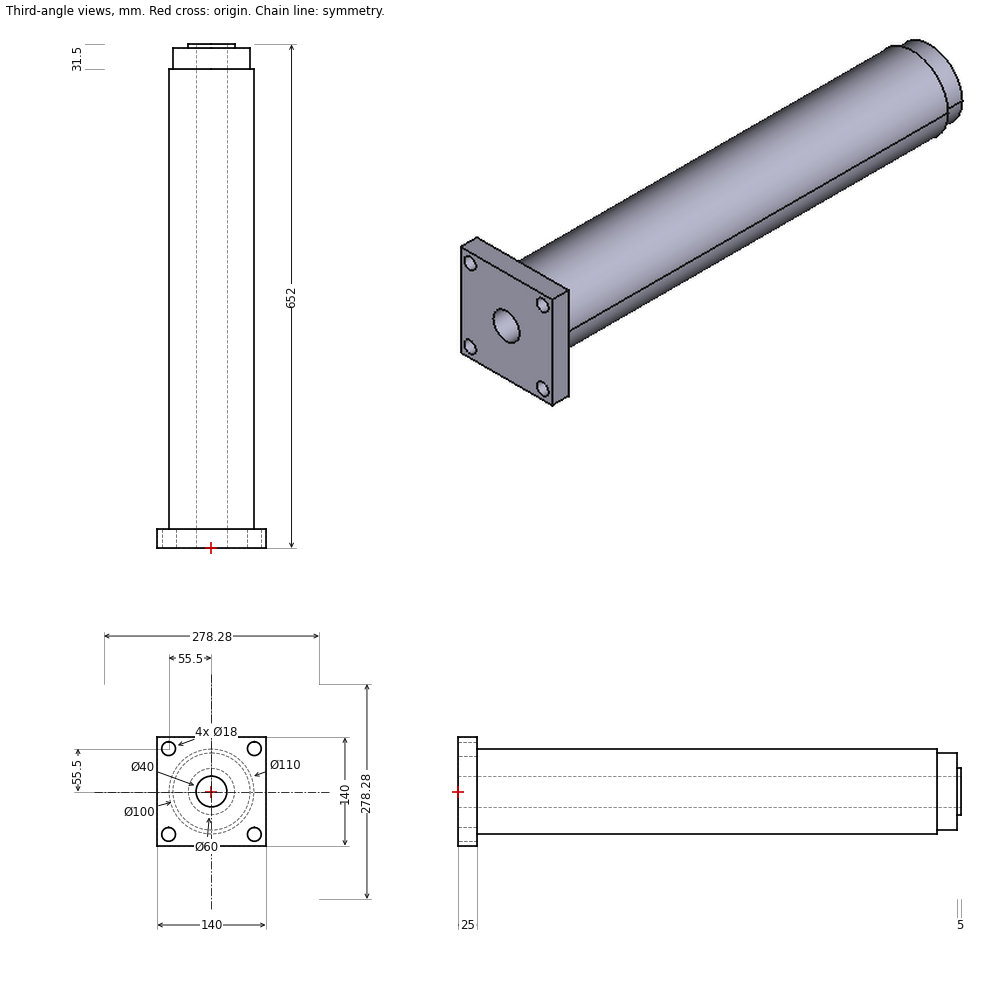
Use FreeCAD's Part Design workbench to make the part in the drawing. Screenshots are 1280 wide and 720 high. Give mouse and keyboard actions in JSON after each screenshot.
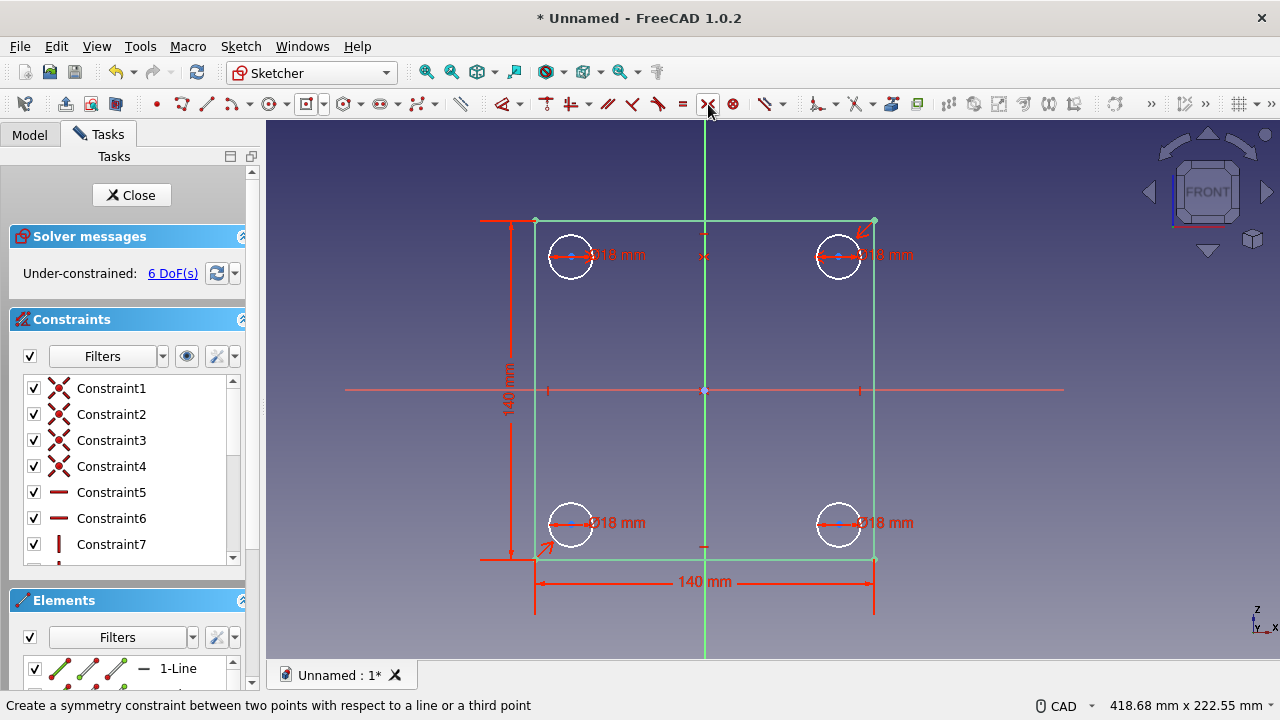
{"action": "left_click", "coordinate": [571, 257]}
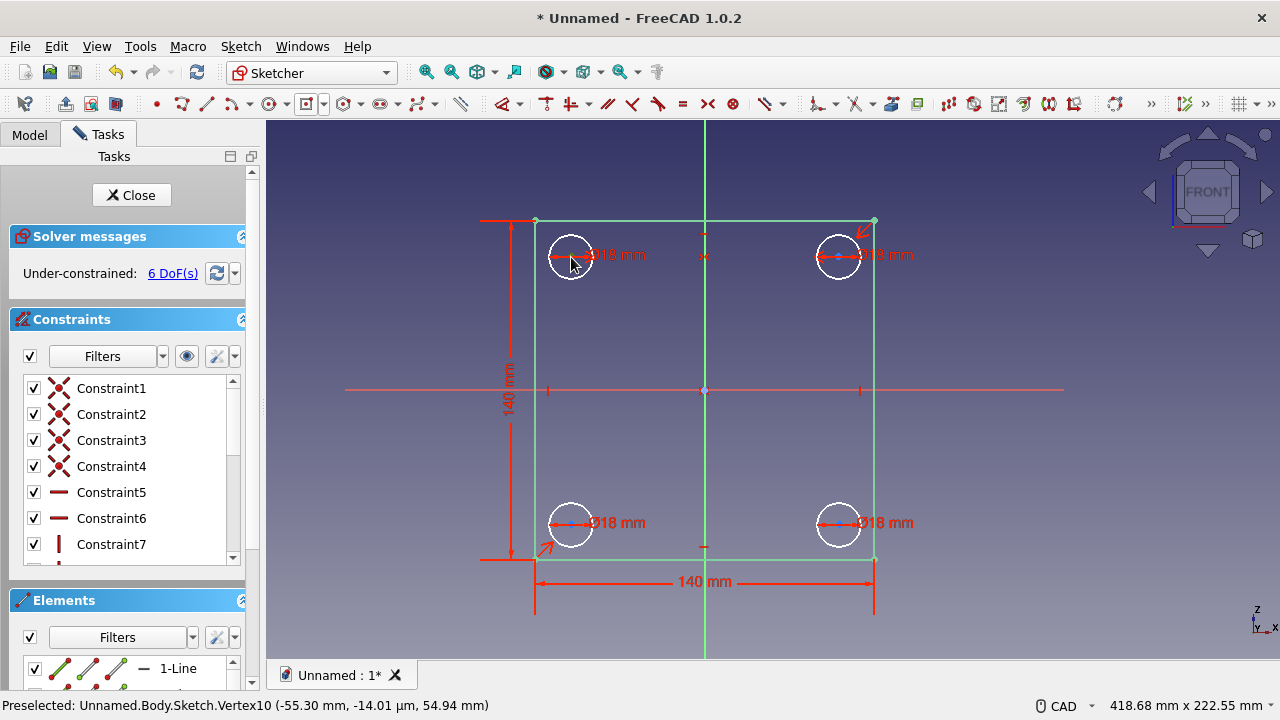
{"action": "left_click", "coordinate": [571, 525]}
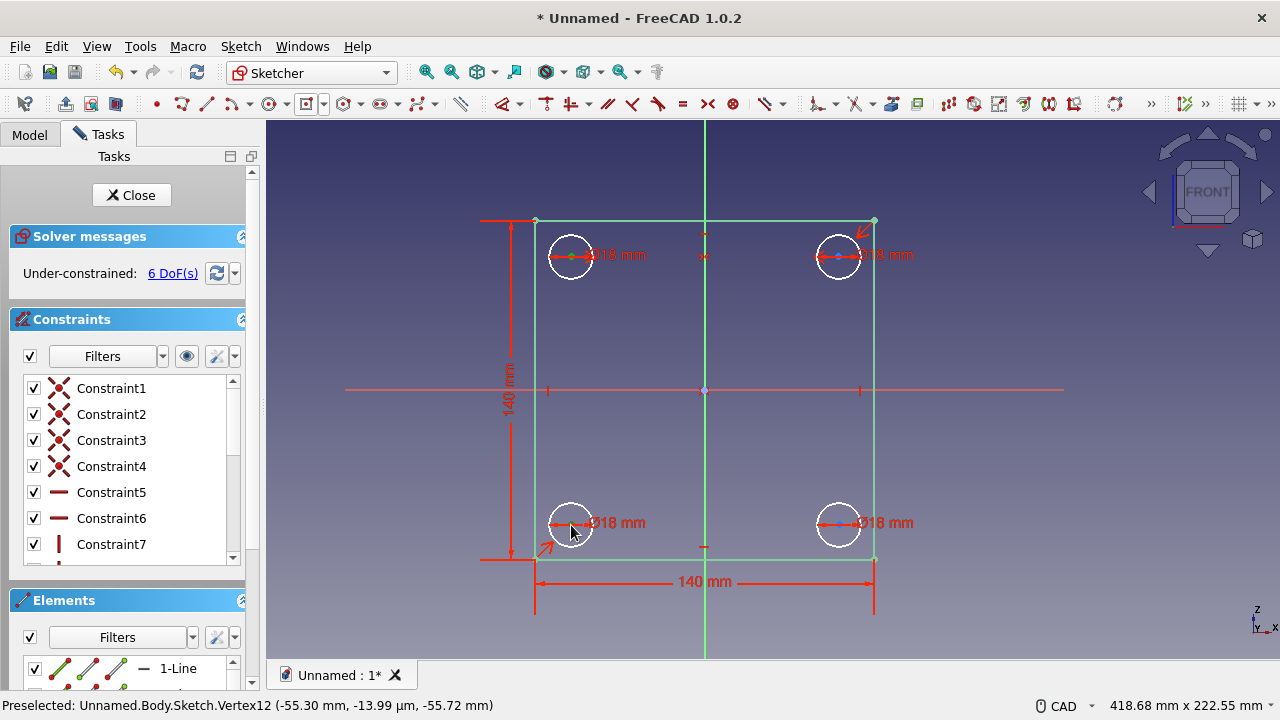
{"action": "left_click", "coordinate": [353, 390]}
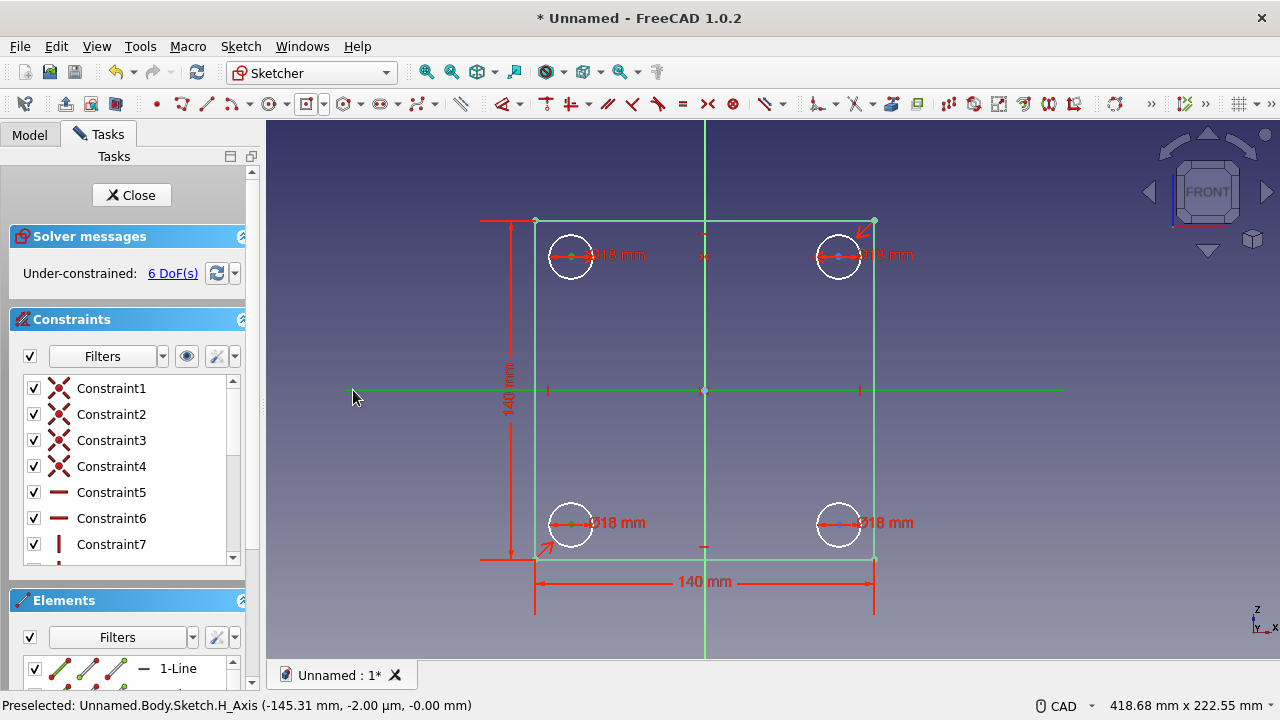
{"action": "left_click", "coordinate": [708, 104]}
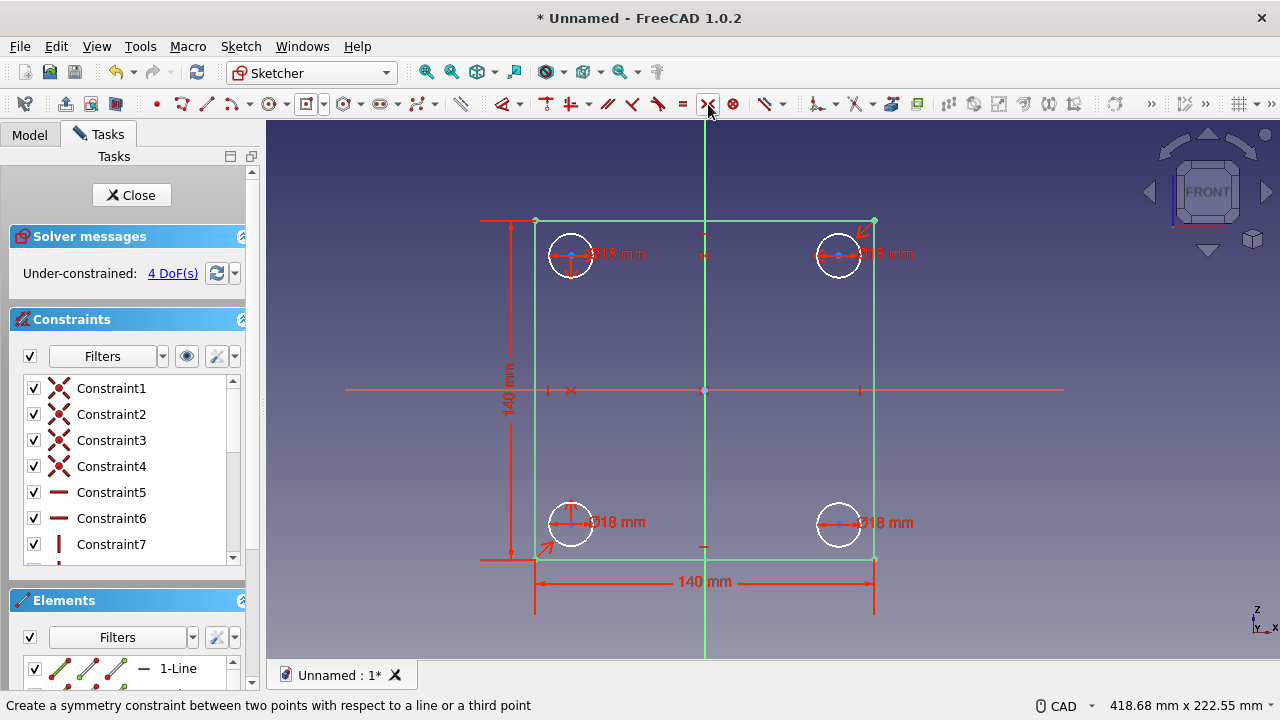
{"action": "left_click", "coordinate": [839, 256]}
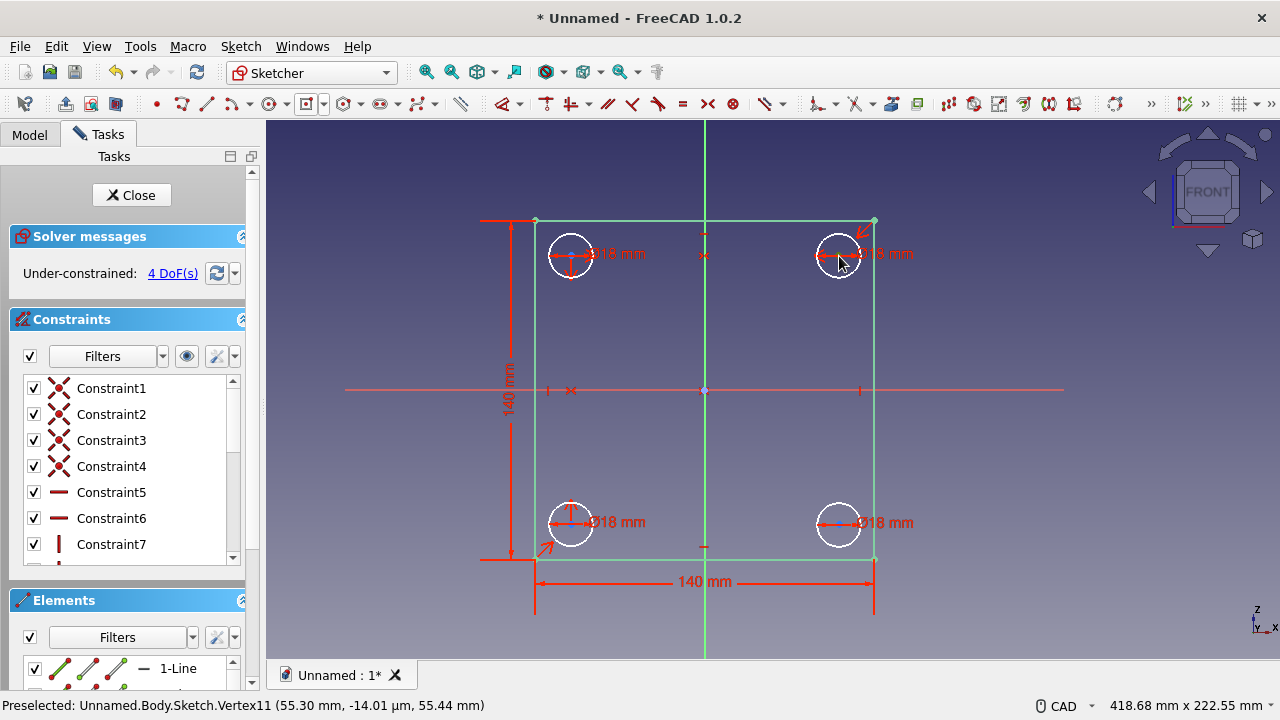
{"action": "left_click", "coordinate": [839, 525]}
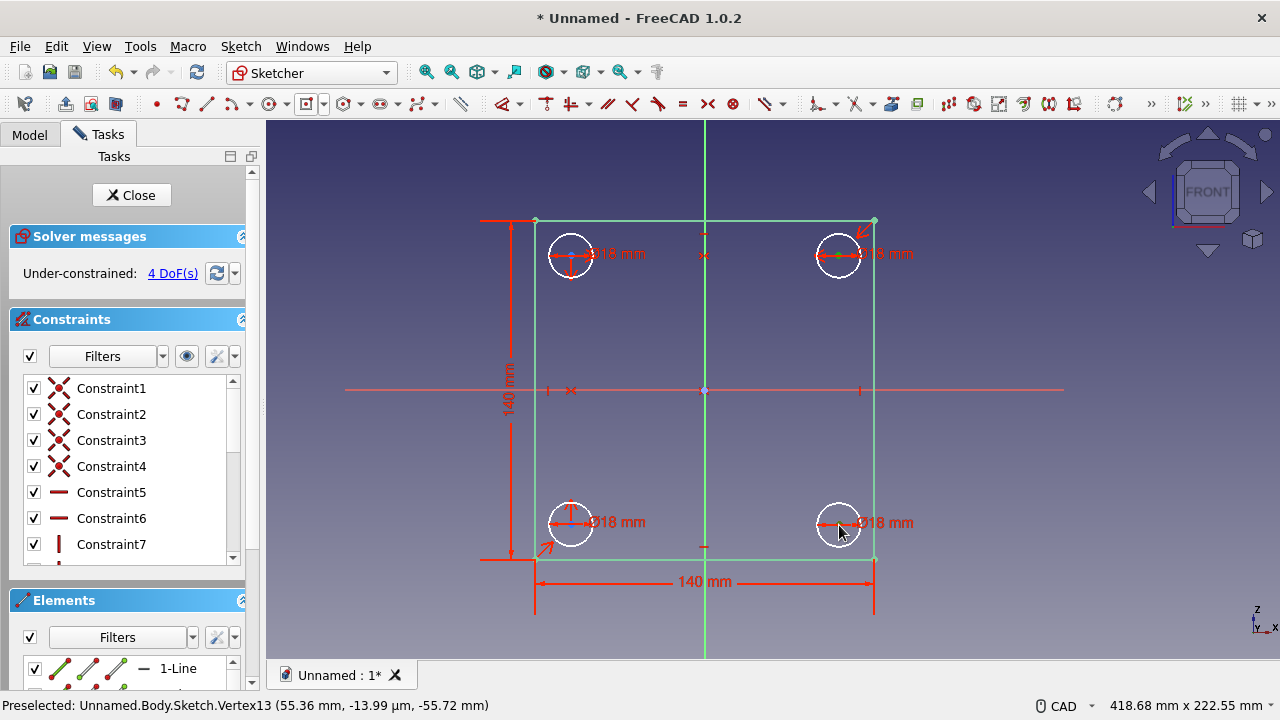
{"action": "left_click", "coordinate": [353, 390]}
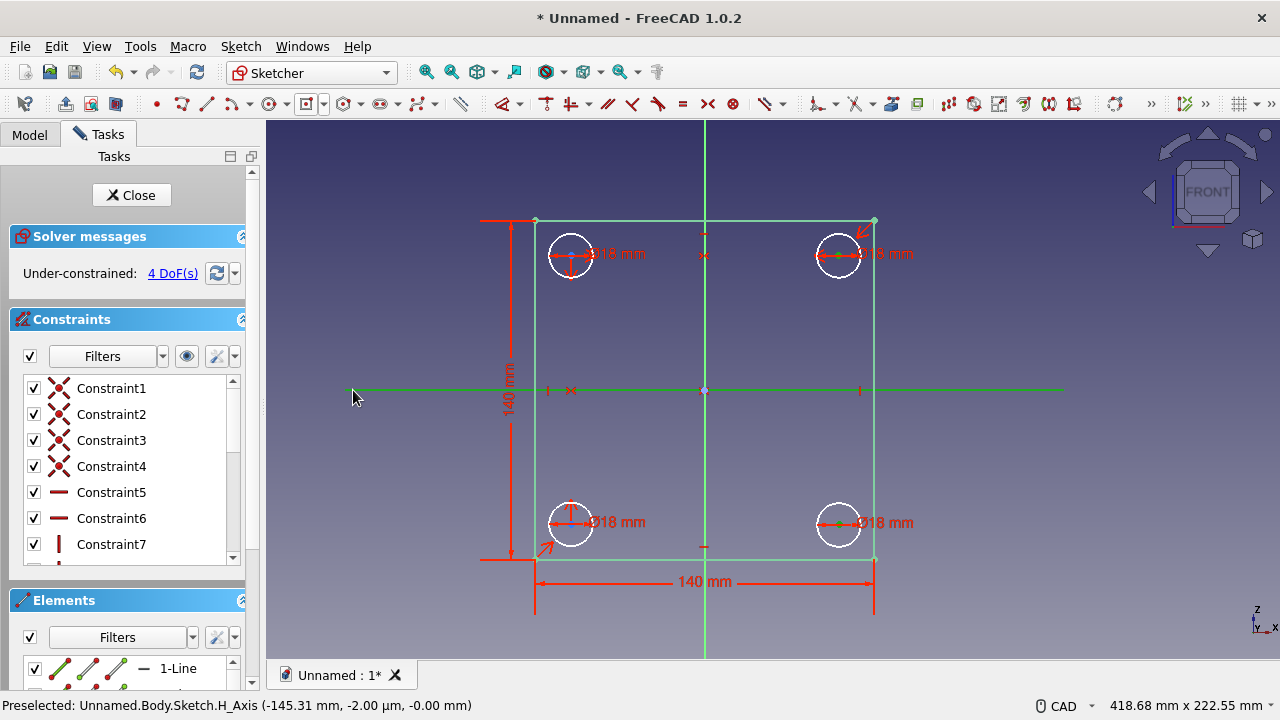
{"action": "left_click", "coordinate": [708, 104]}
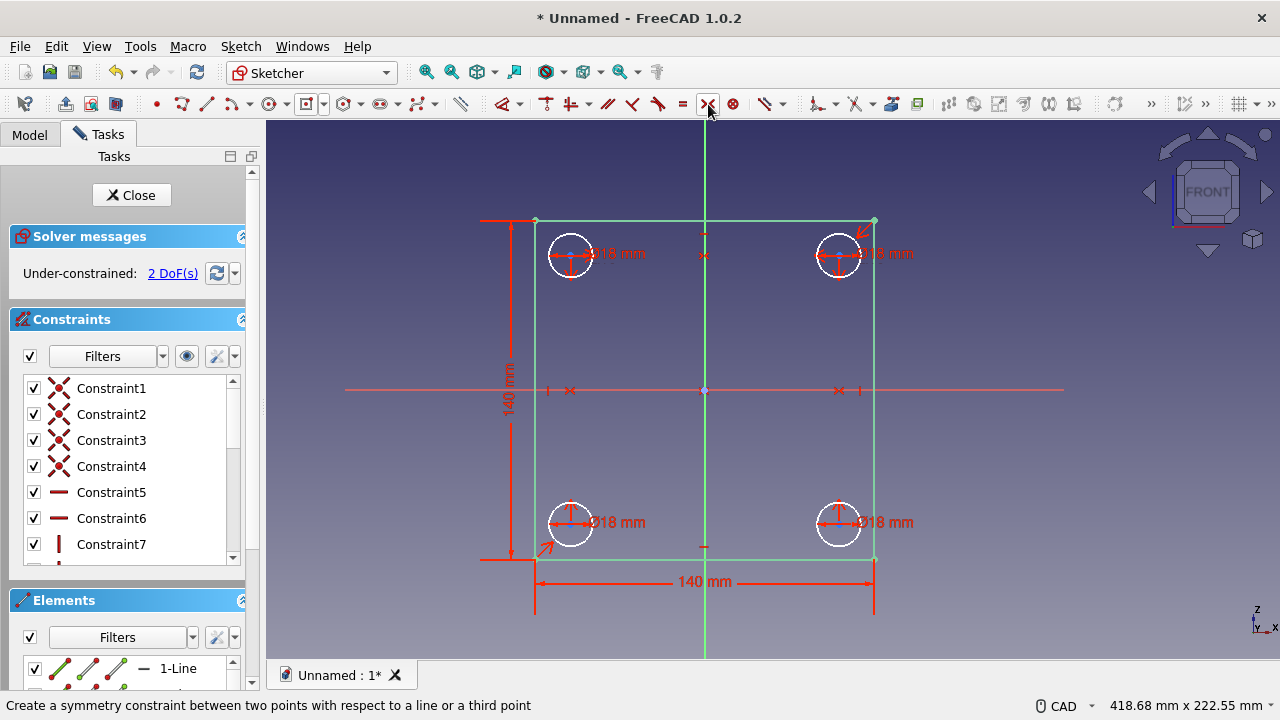
{"action": "left_click", "coordinate": [502, 104]}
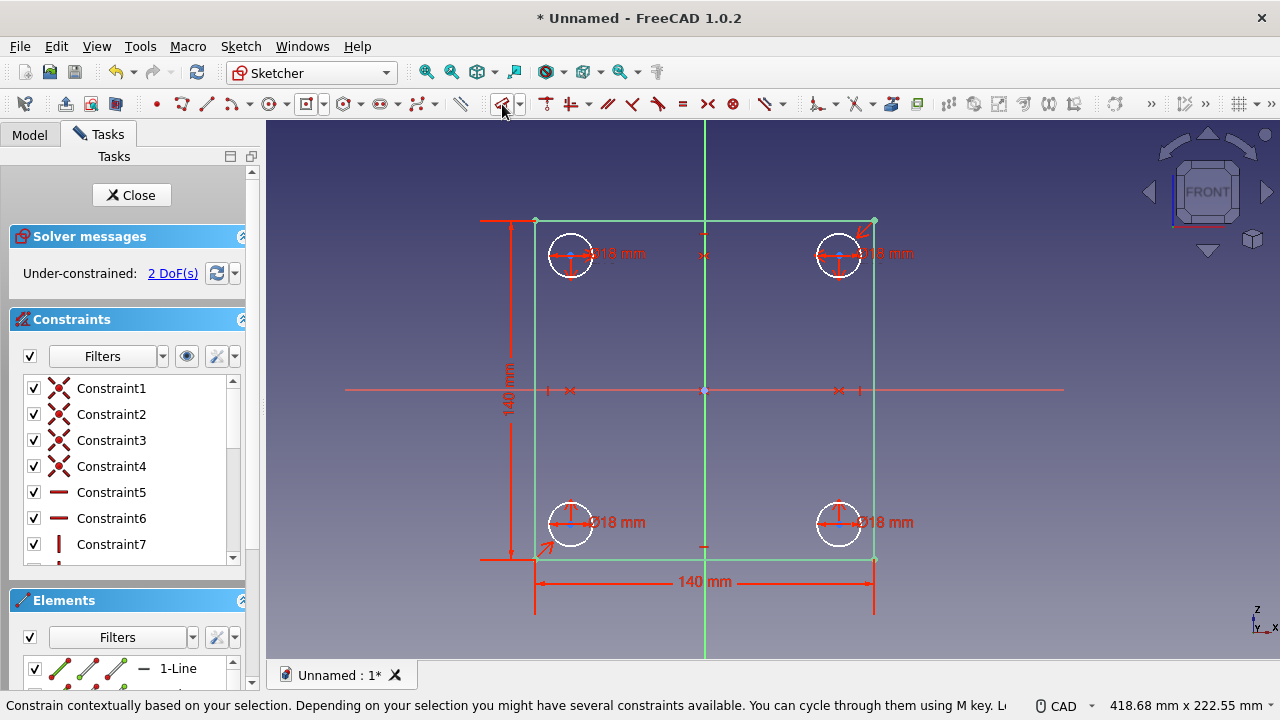
{"action": "left_click", "coordinate": [571, 256]}
{"action": "left_click", "coordinate": [638, 424]}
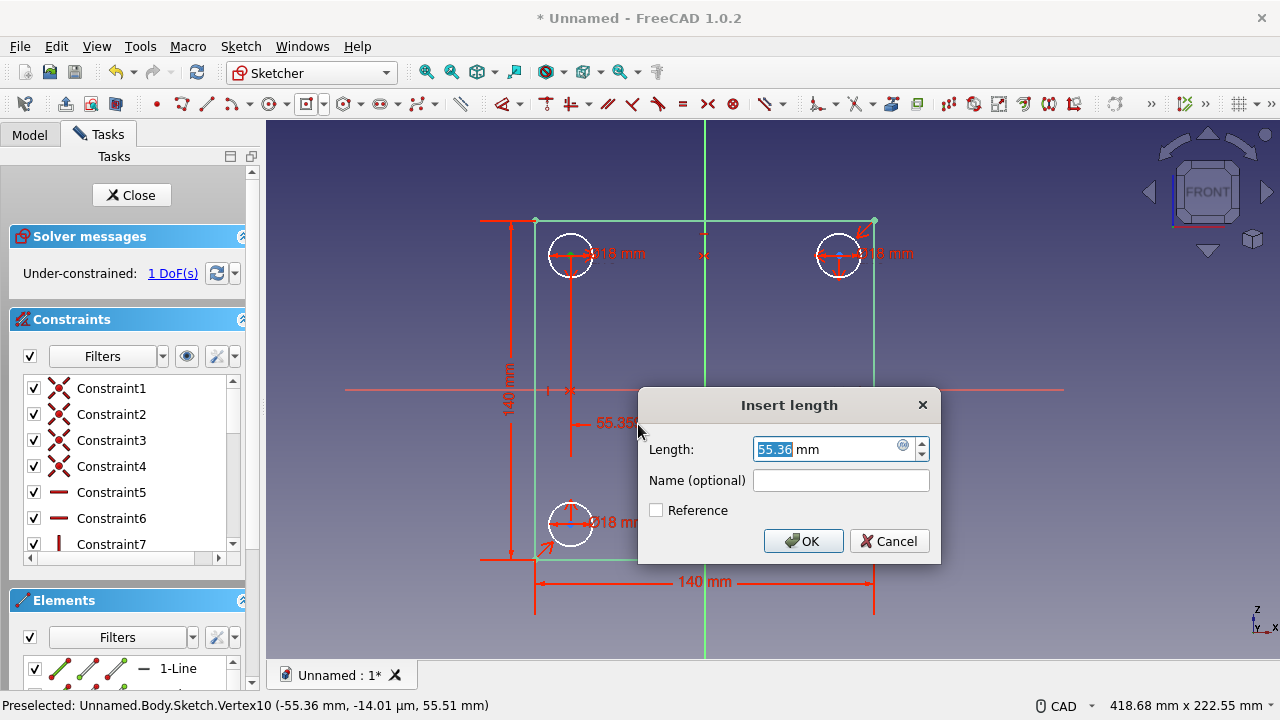
{"action": "type", "text": "55.5"}
{"action": "key", "text": "Return"}